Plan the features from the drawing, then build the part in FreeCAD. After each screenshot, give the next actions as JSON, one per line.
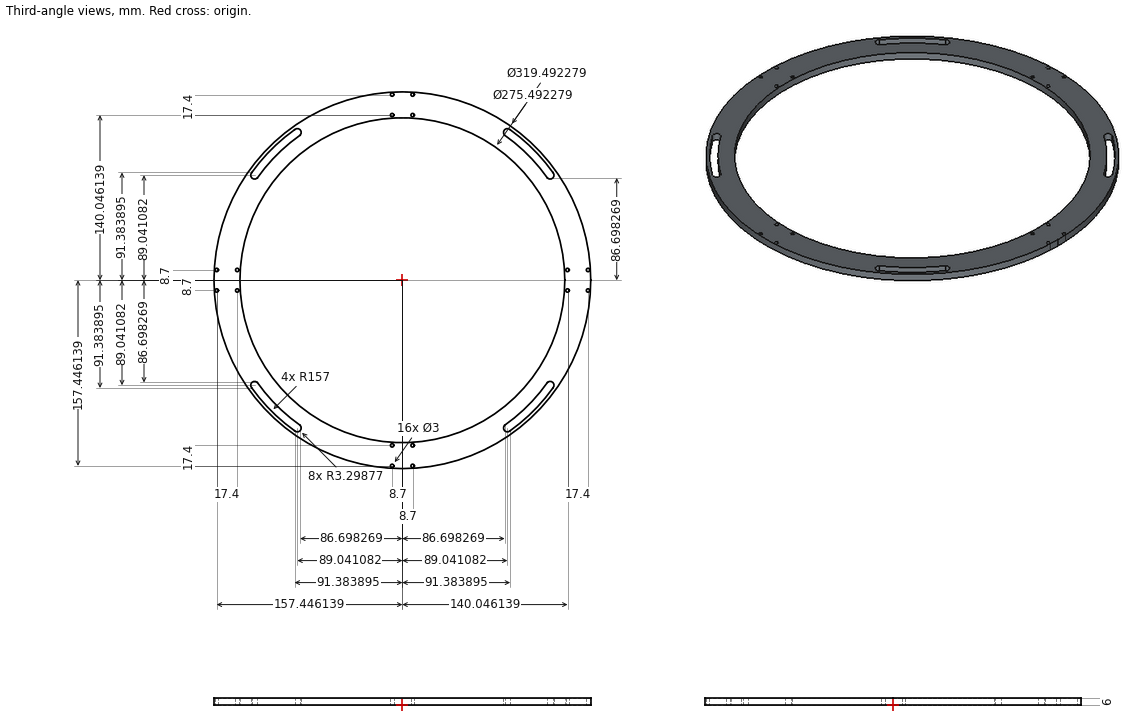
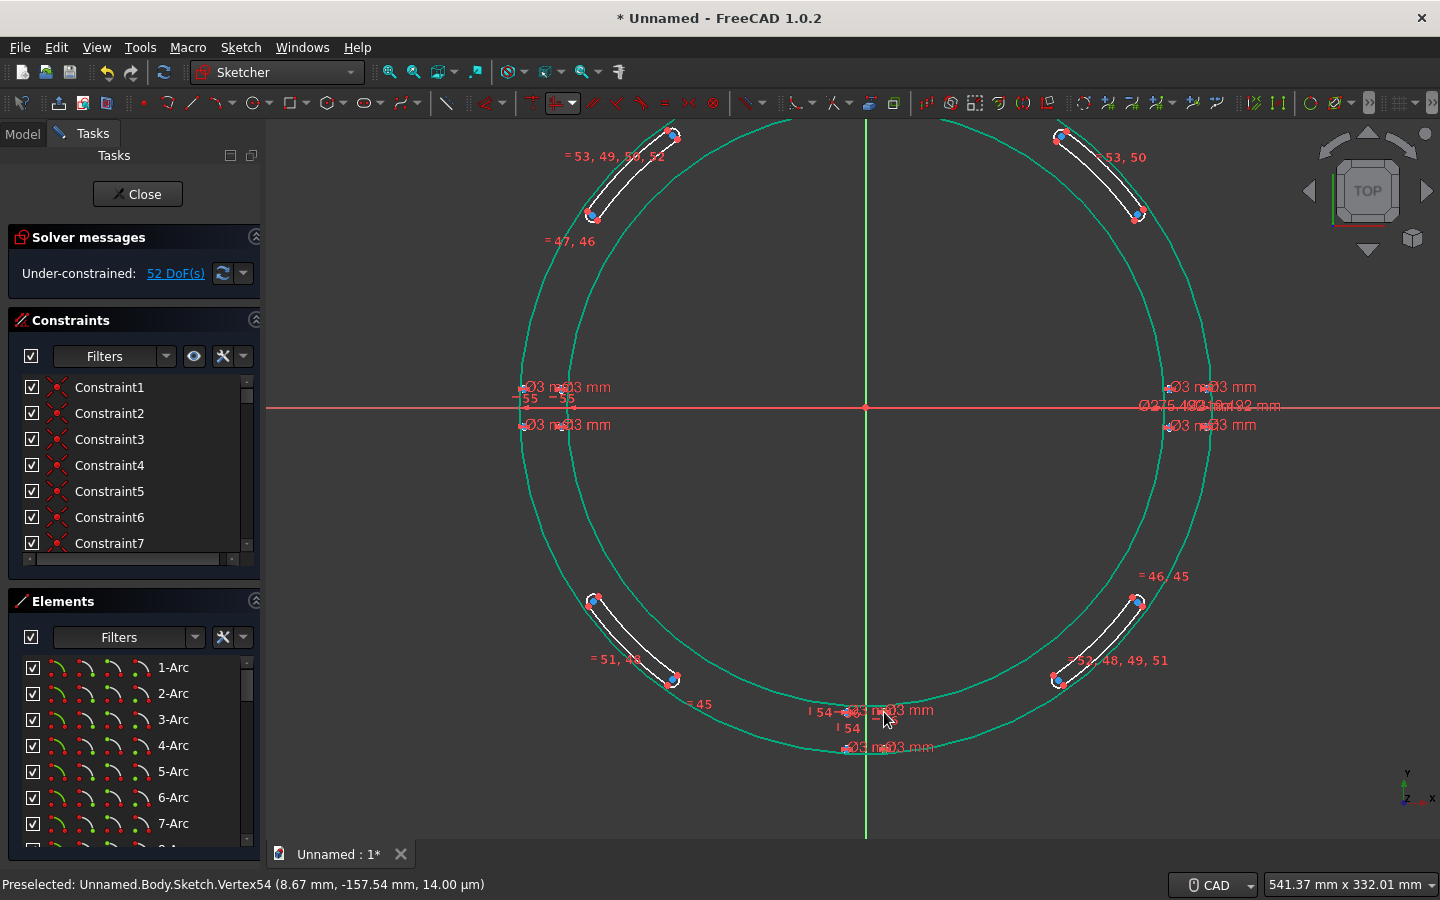
{"action": "key", "text": "v"}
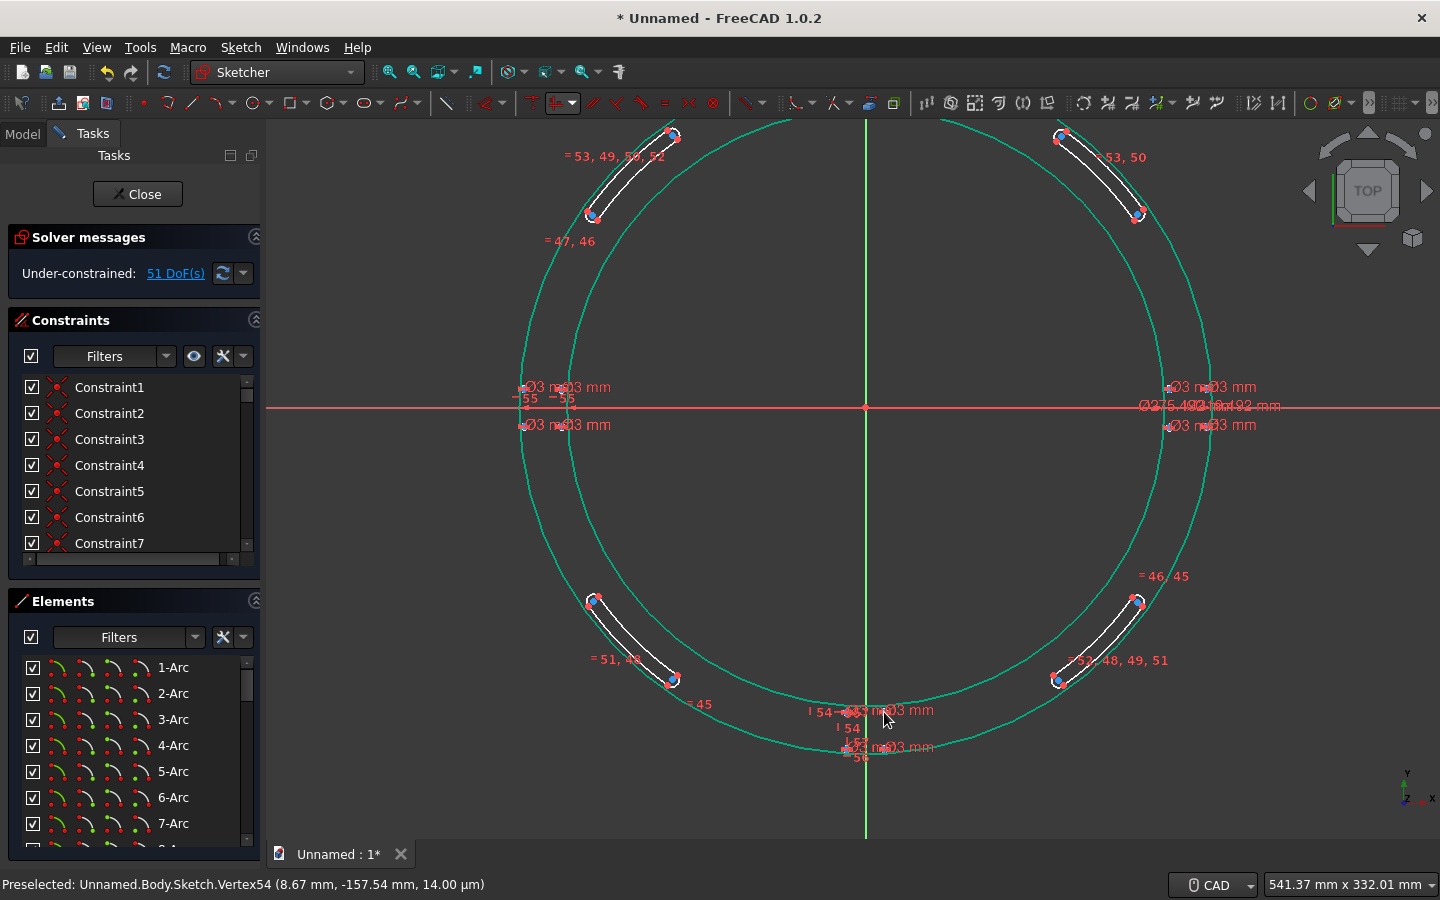
{"action": "scroll", "coordinate": [847, 712], "scroll_direction": "up", "scroll_amount": 4}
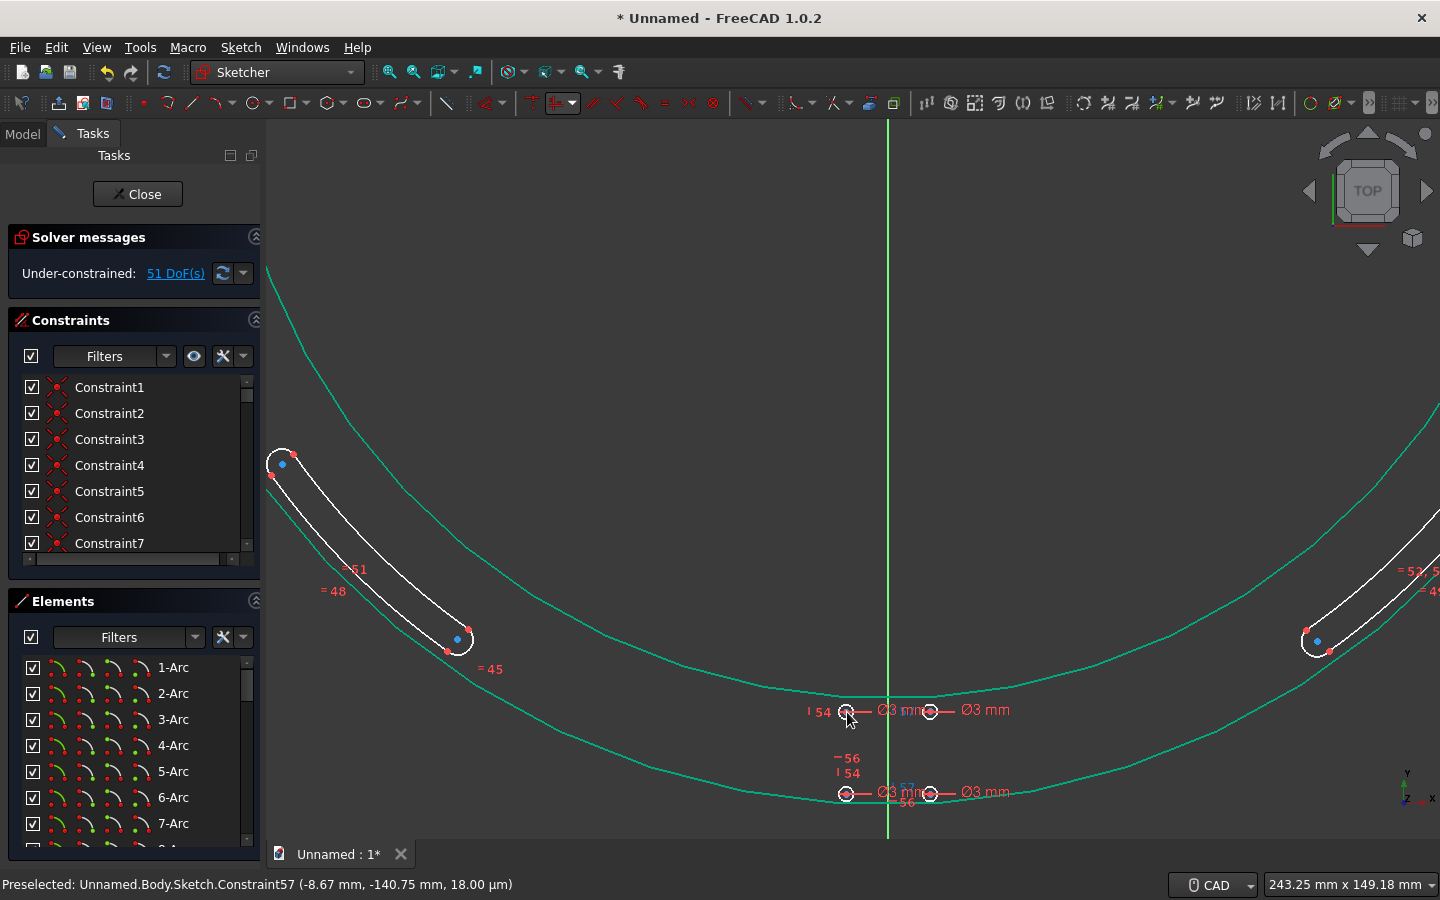
{"action": "left_click", "coordinate": [846, 712]}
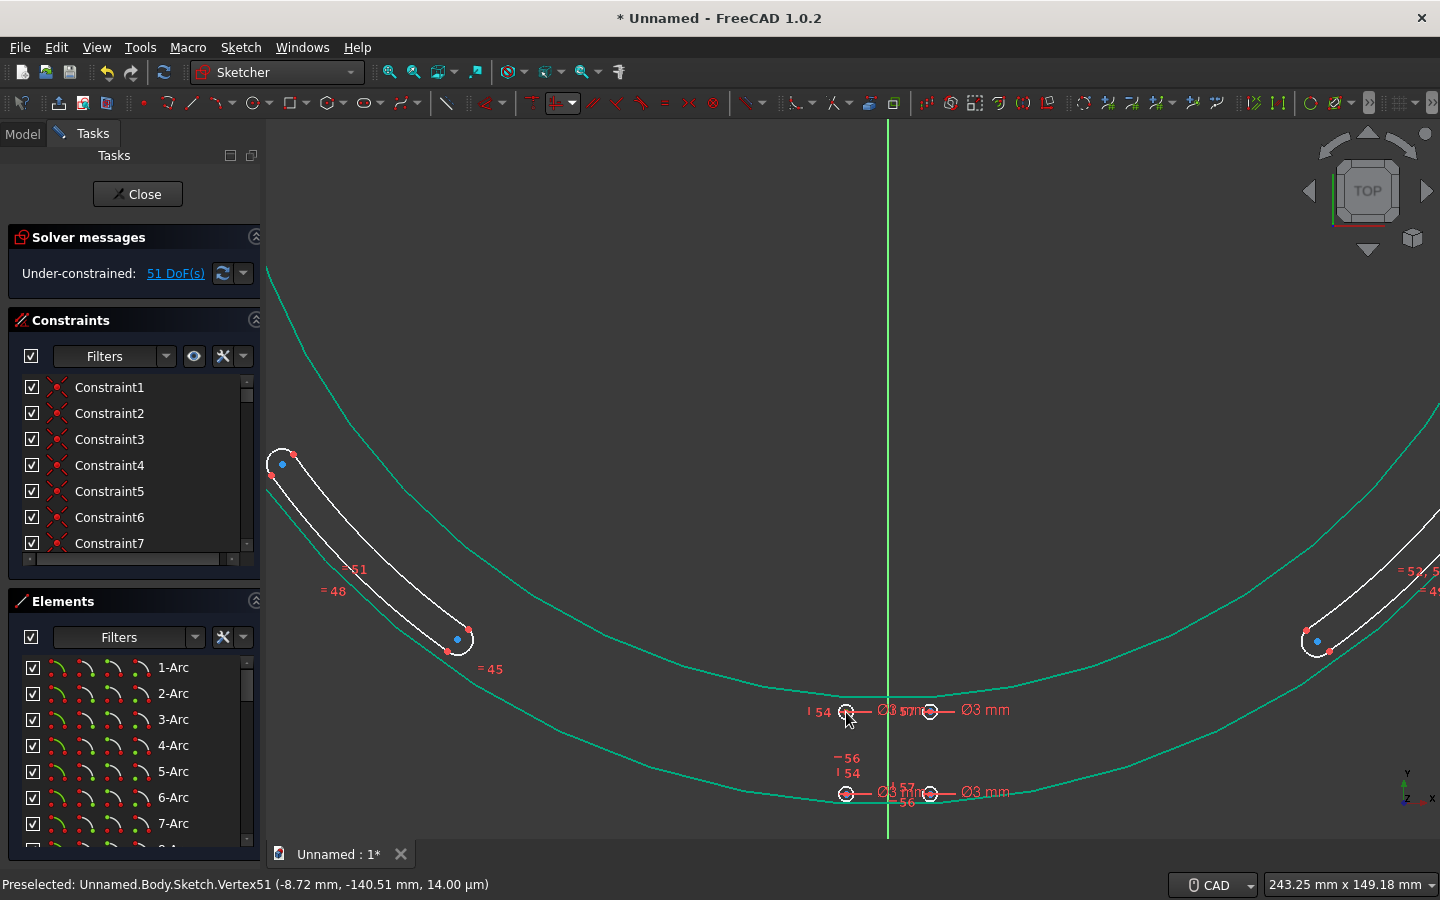
{"action": "left_click", "coordinate": [930, 712]}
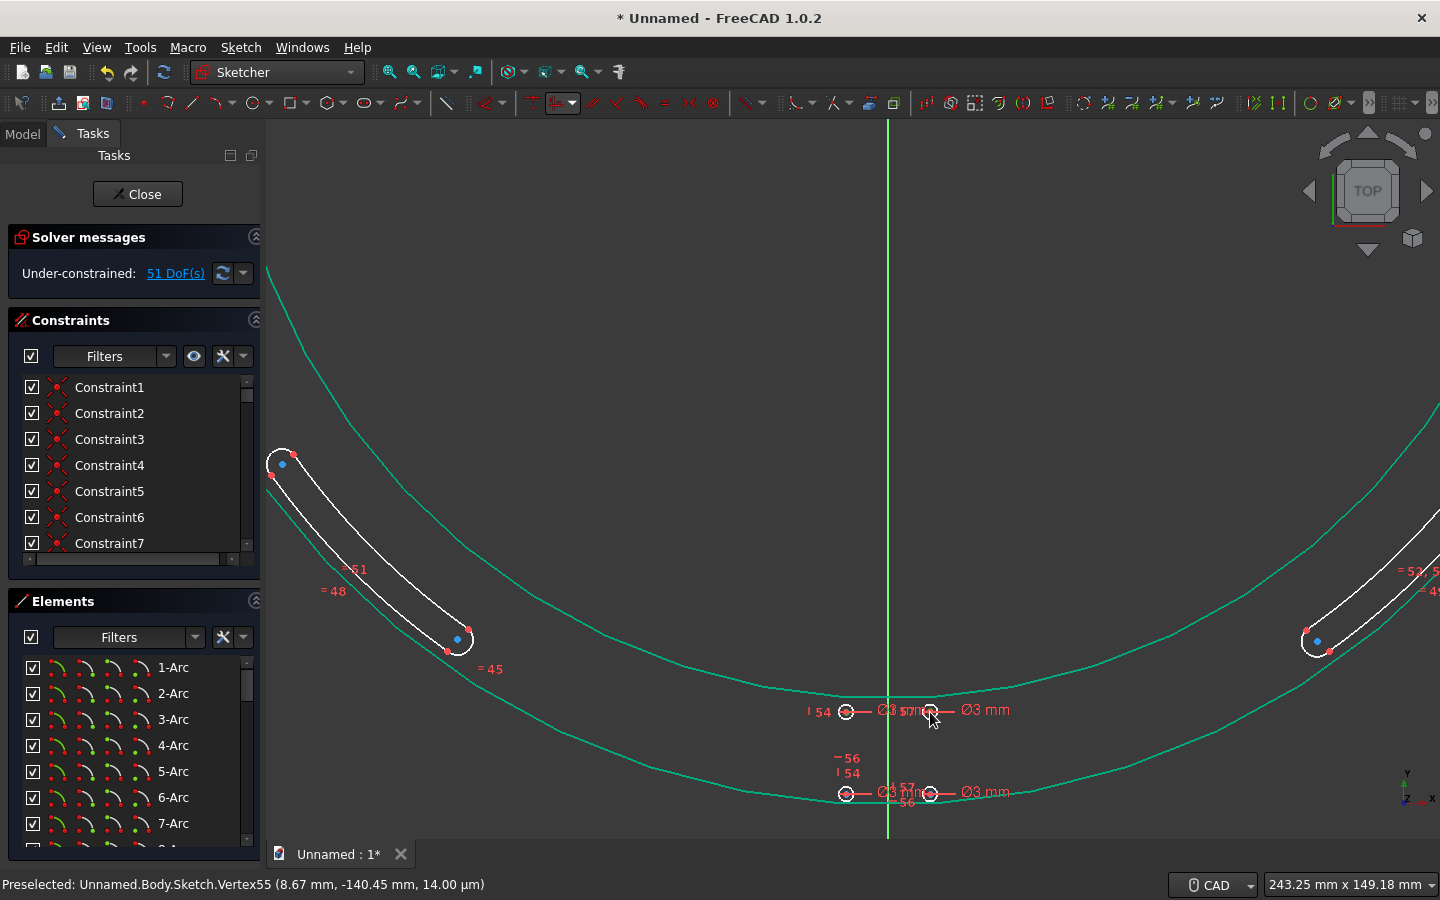
{"action": "key", "text": "h"}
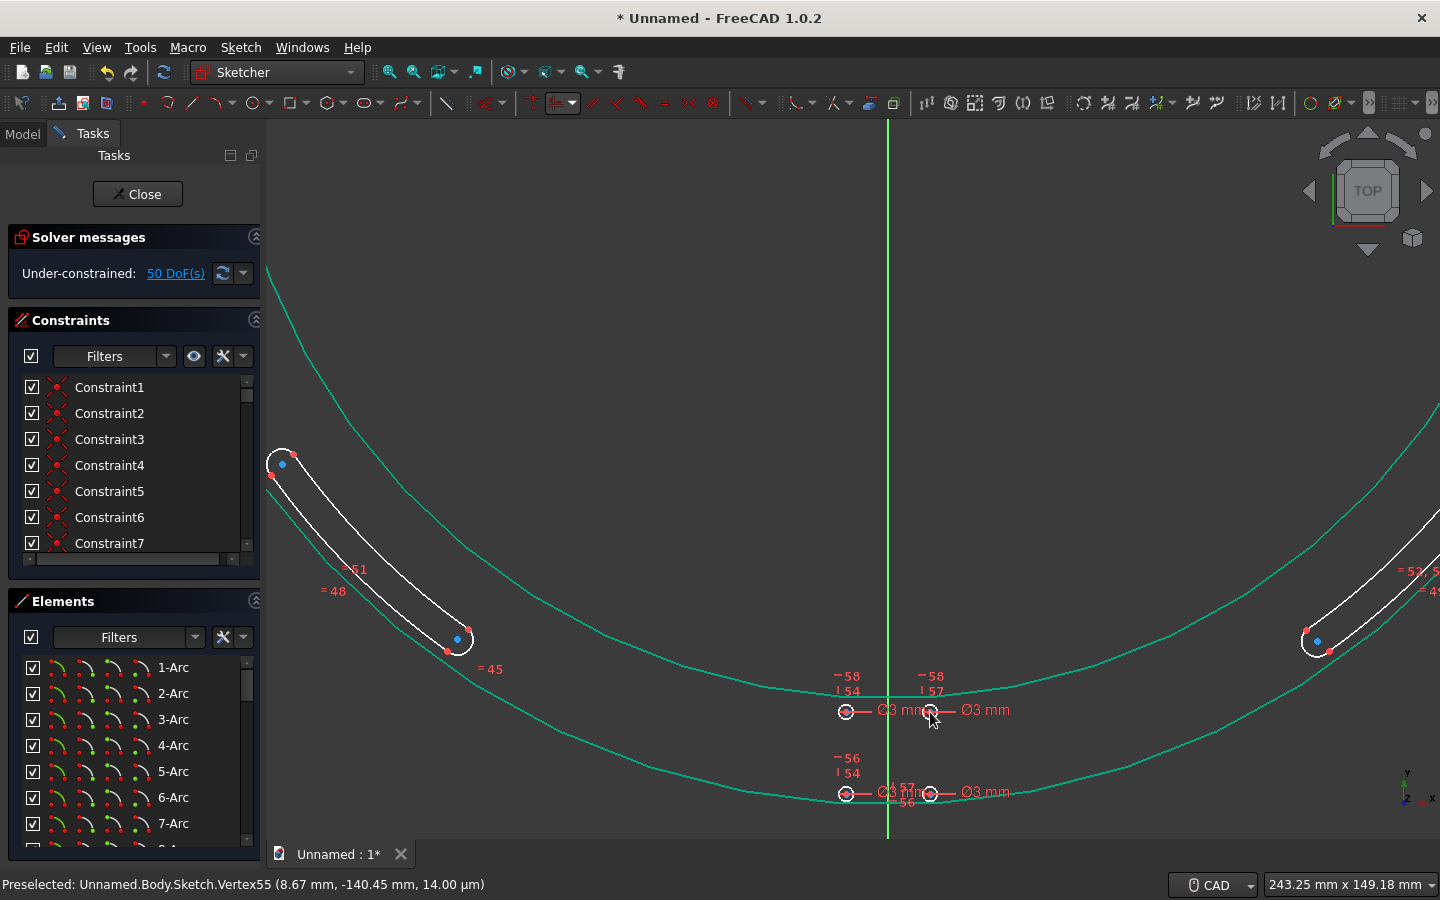
{"action": "scroll", "coordinate": [740, 671], "scroll_direction": "down", "scroll_amount": 6}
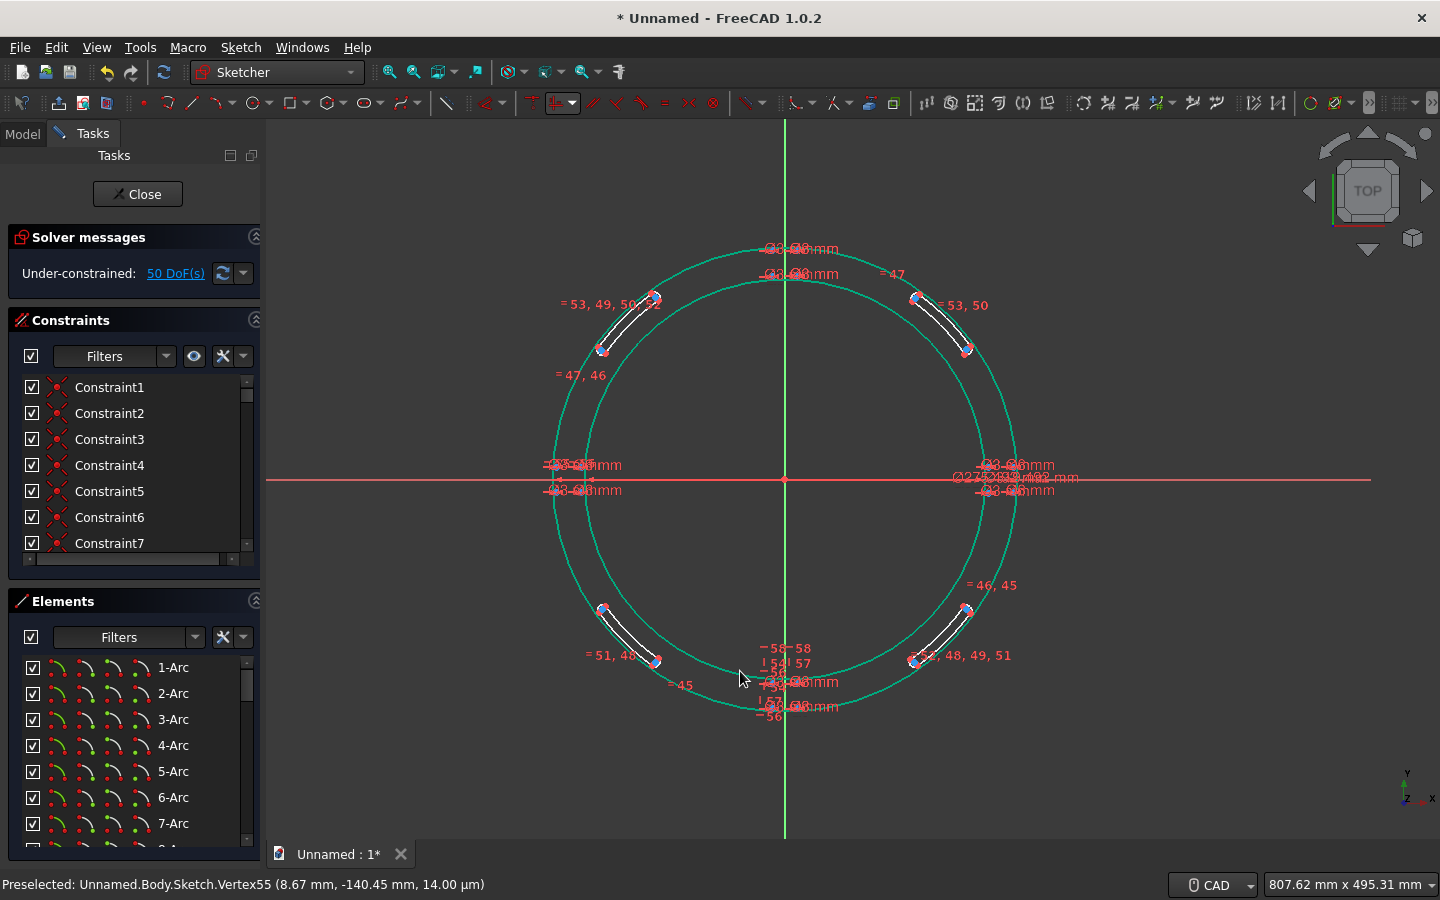
{"action": "left_click", "coordinate": [988, 493]}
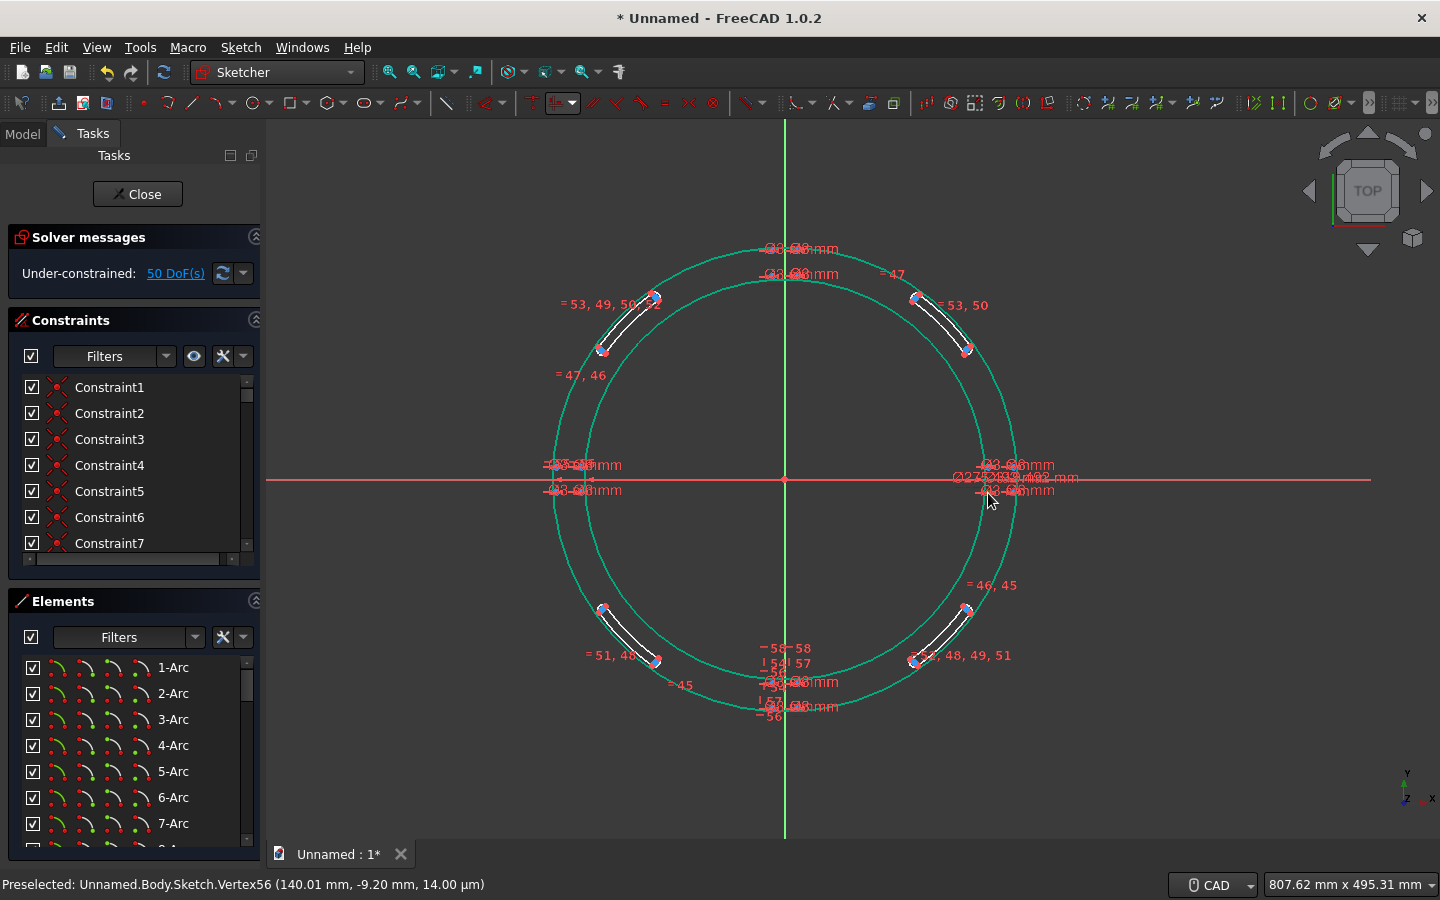
{"action": "left_click", "coordinate": [1014, 492]}